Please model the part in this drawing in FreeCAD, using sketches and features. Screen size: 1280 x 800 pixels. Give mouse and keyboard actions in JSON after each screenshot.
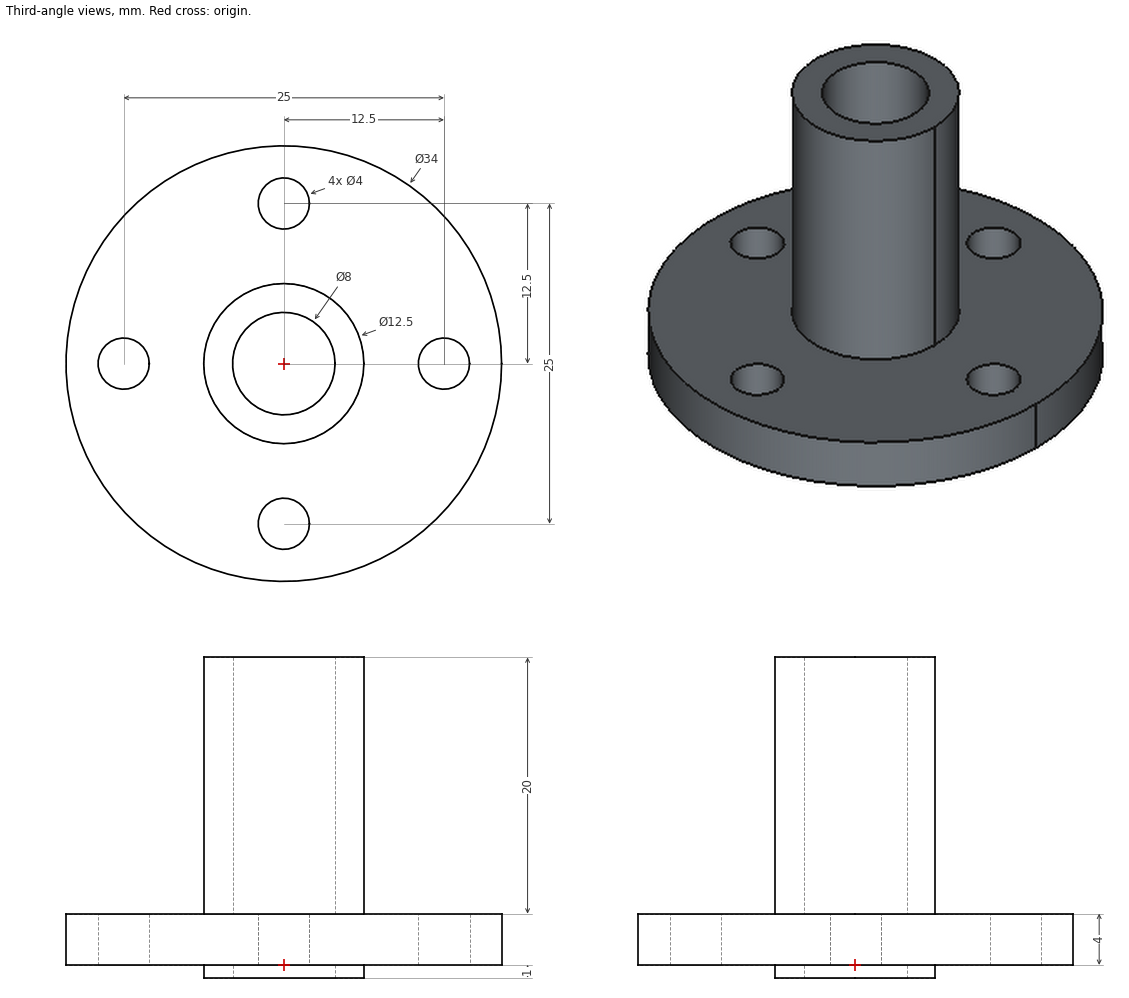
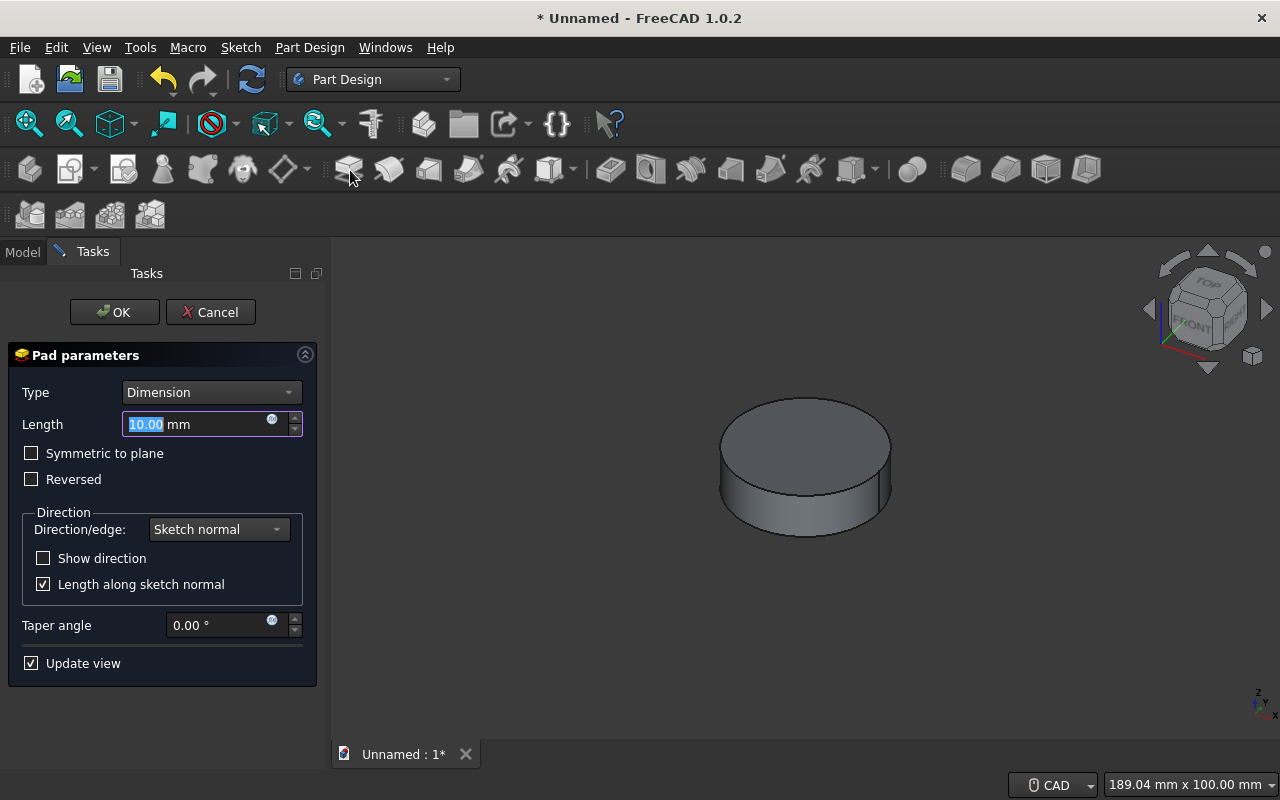
{"action": "type", "text": "4"}
{"action": "key", "text": "Tab"}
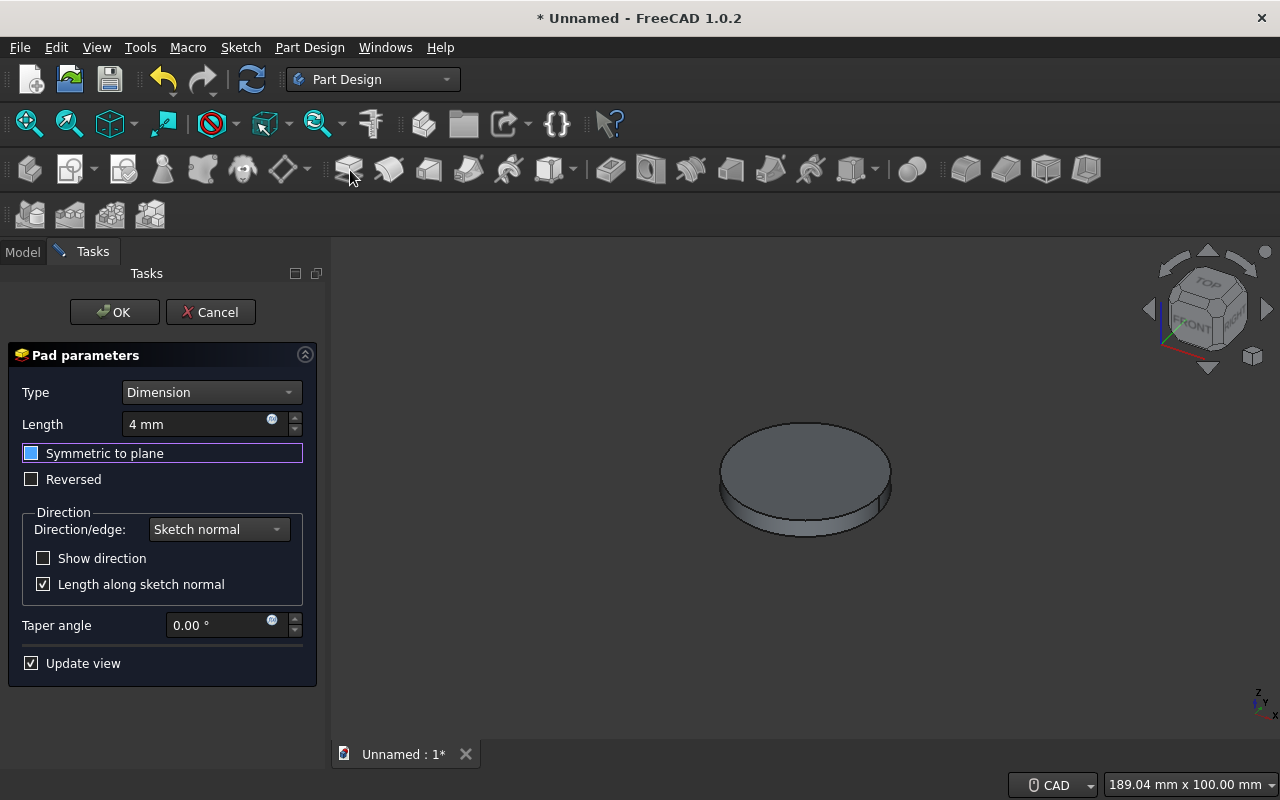
{"action": "left_click", "coordinate": [115, 312]}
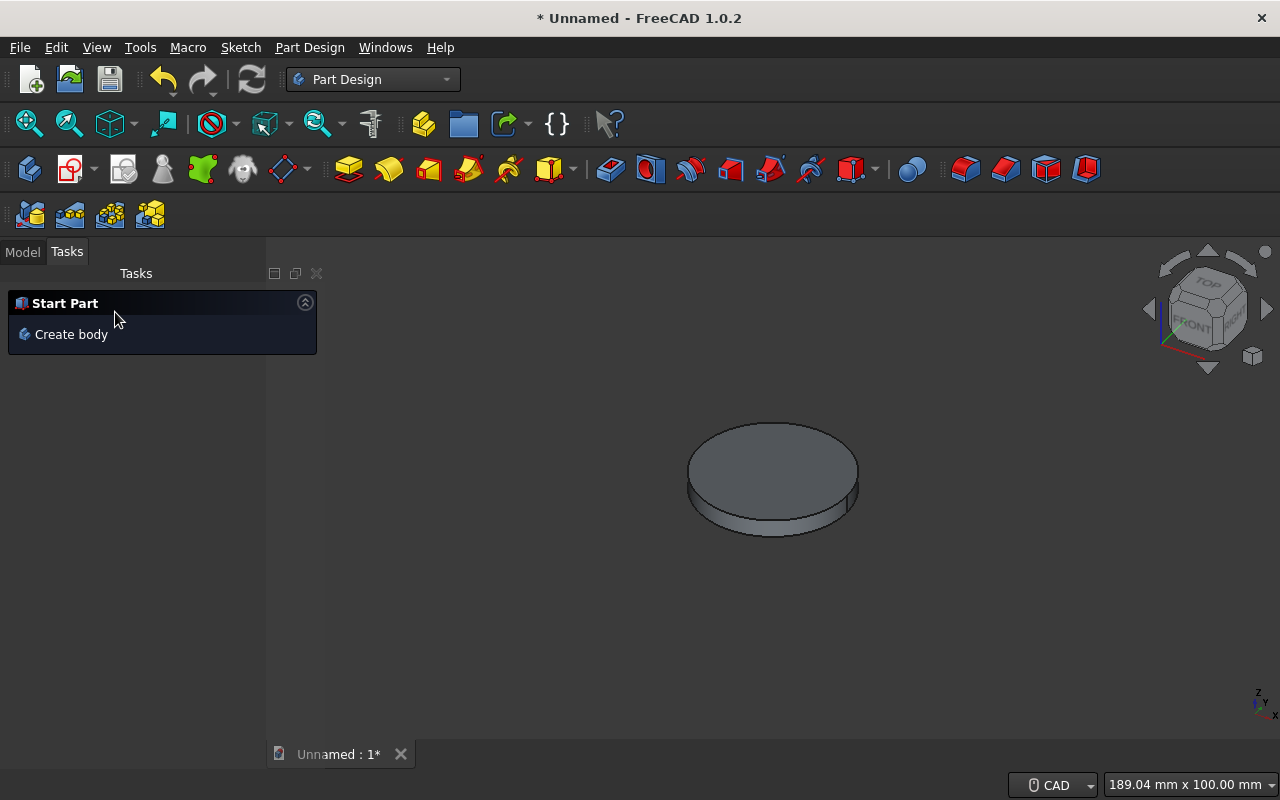
{"action": "left_click", "coordinate": [30, 124]}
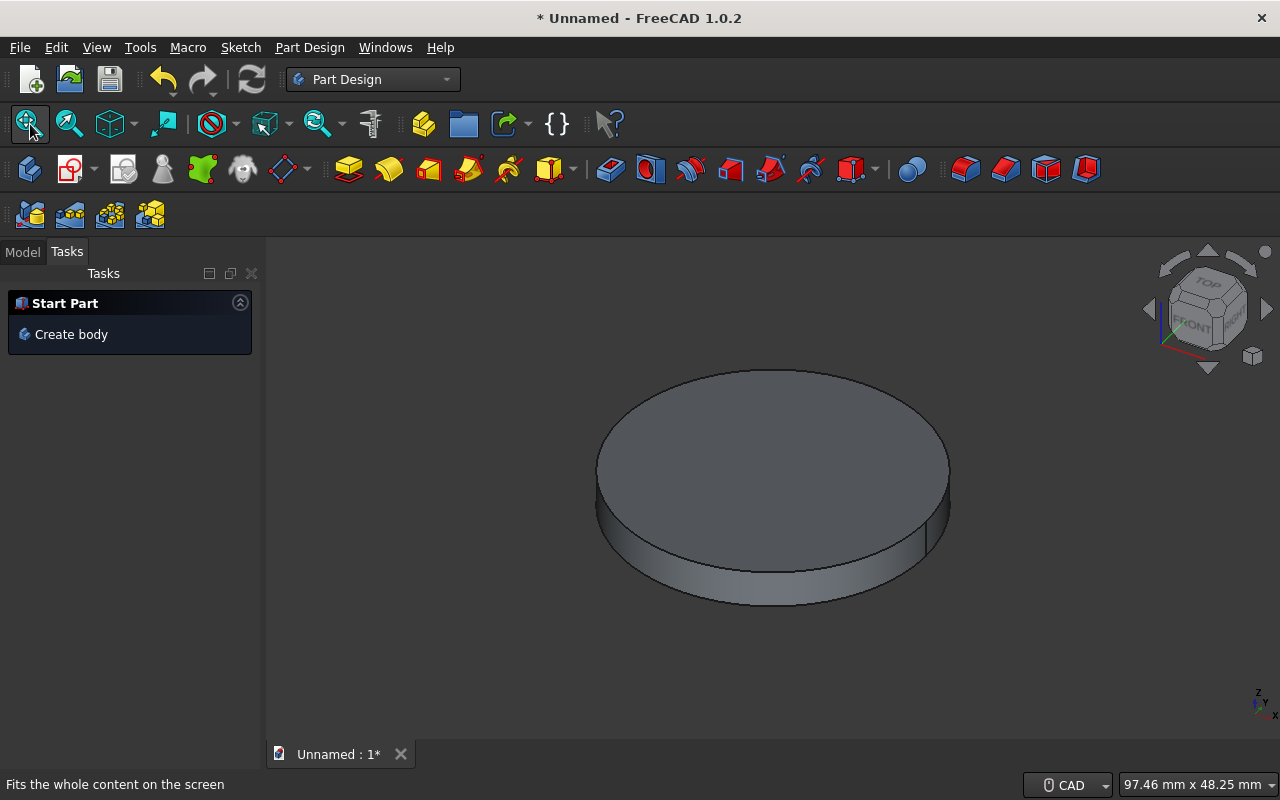
{"action": "left_click", "coordinate": [773, 470]}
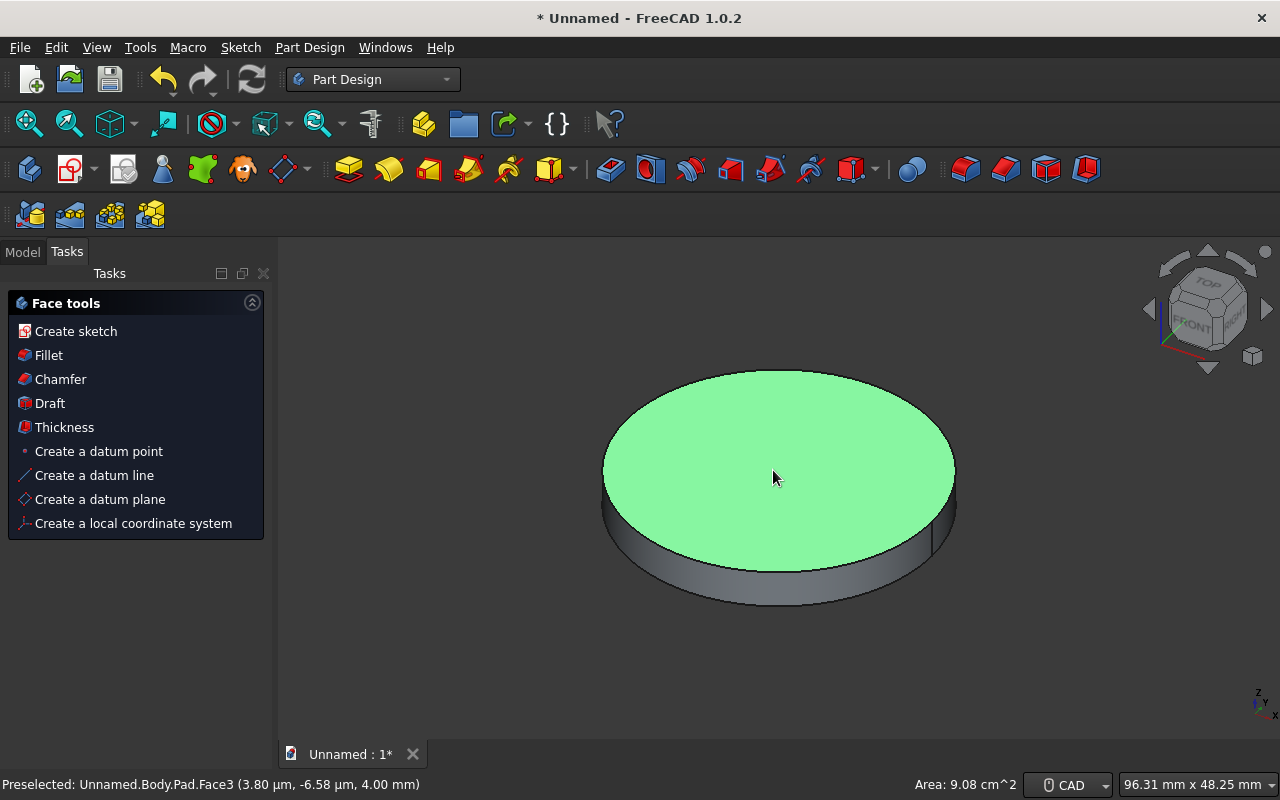
{"action": "left_click", "coordinate": [70, 170]}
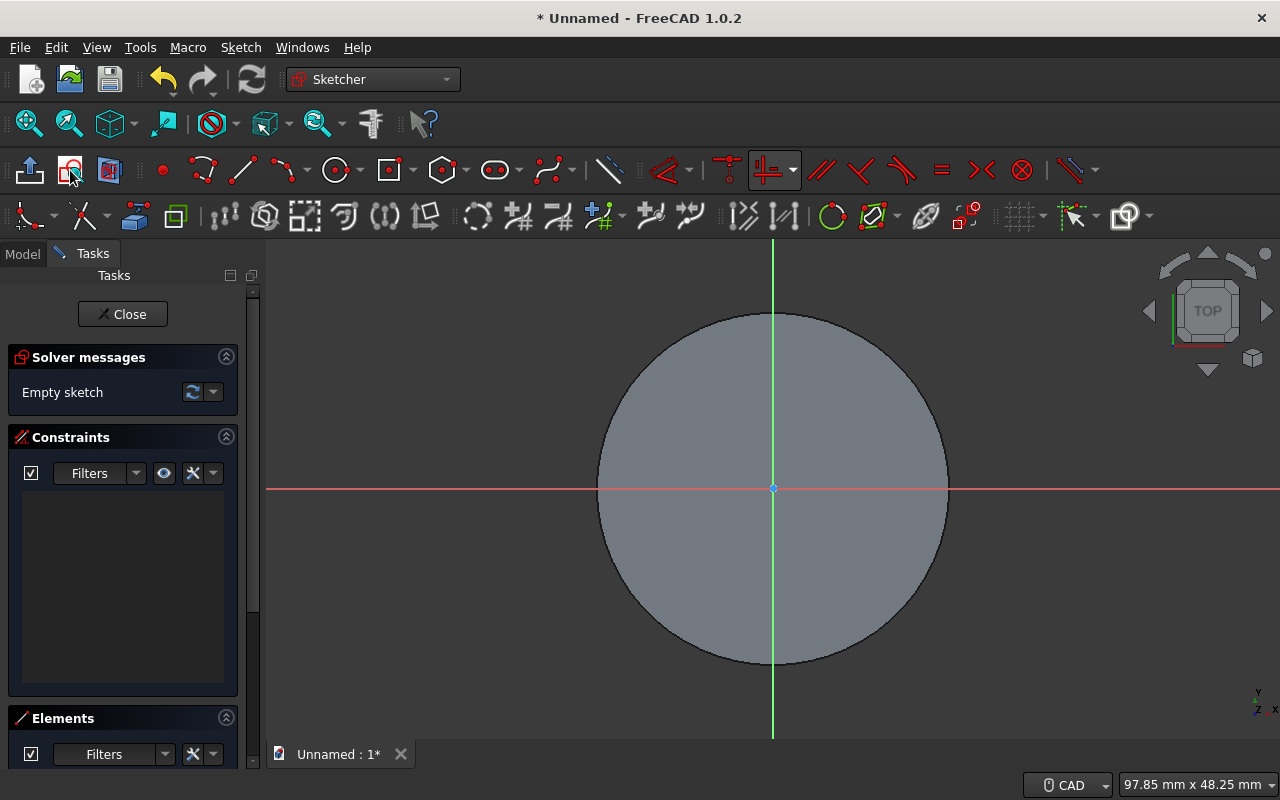
{"action": "scroll", "coordinate": [829, 489], "scroll_direction": "up", "scroll_amount": 4}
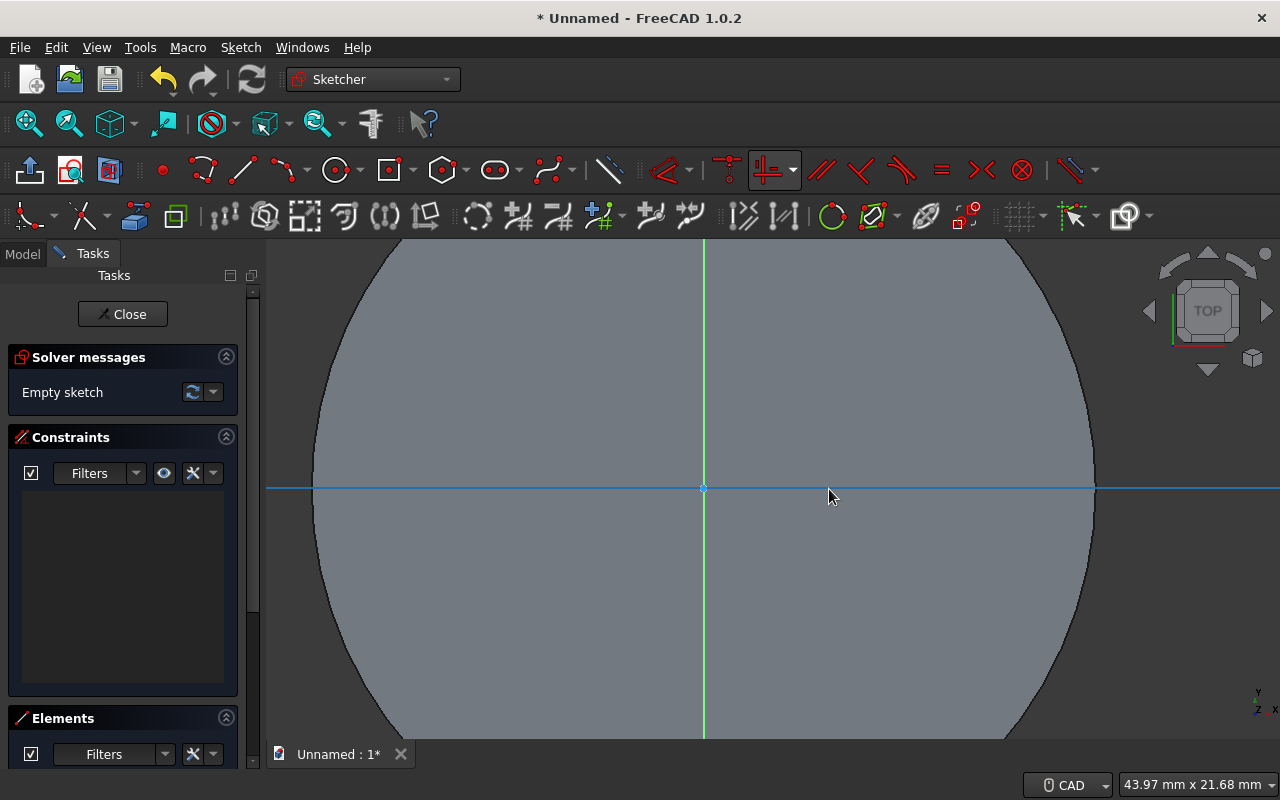
{"action": "left_click", "coordinate": [336, 170]}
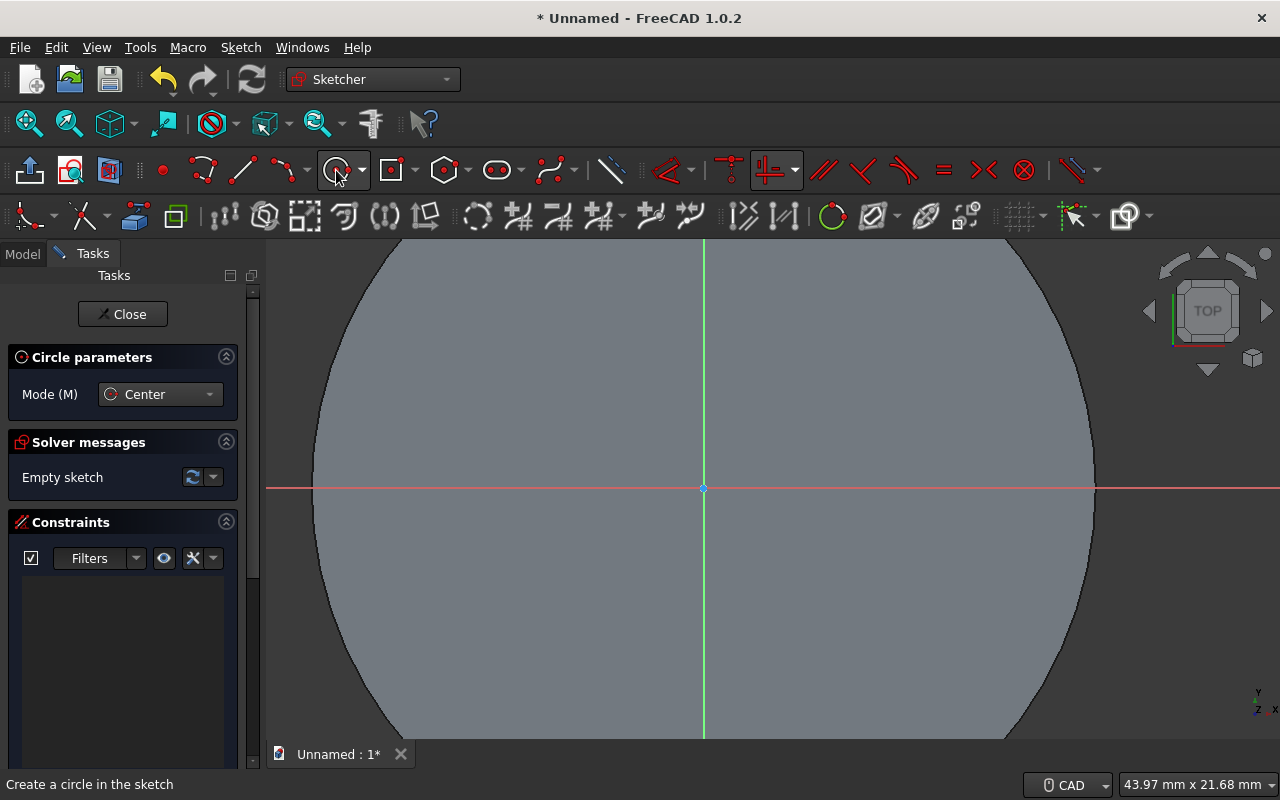
{"action": "left_click", "coordinate": [704, 488]}
{"action": "mouse_move", "coordinate": [806, 386]}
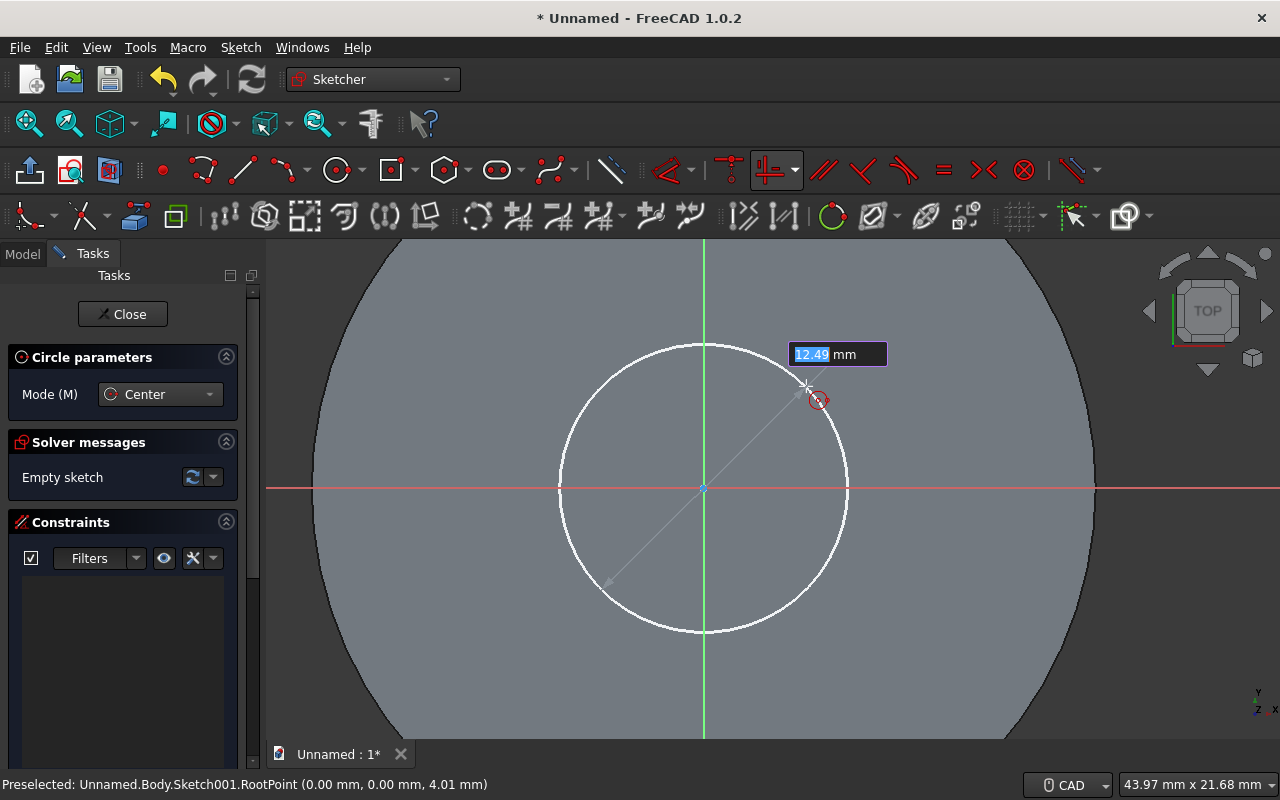
{"action": "type", "text": "12.5"}
{"action": "key", "text": "Return"}